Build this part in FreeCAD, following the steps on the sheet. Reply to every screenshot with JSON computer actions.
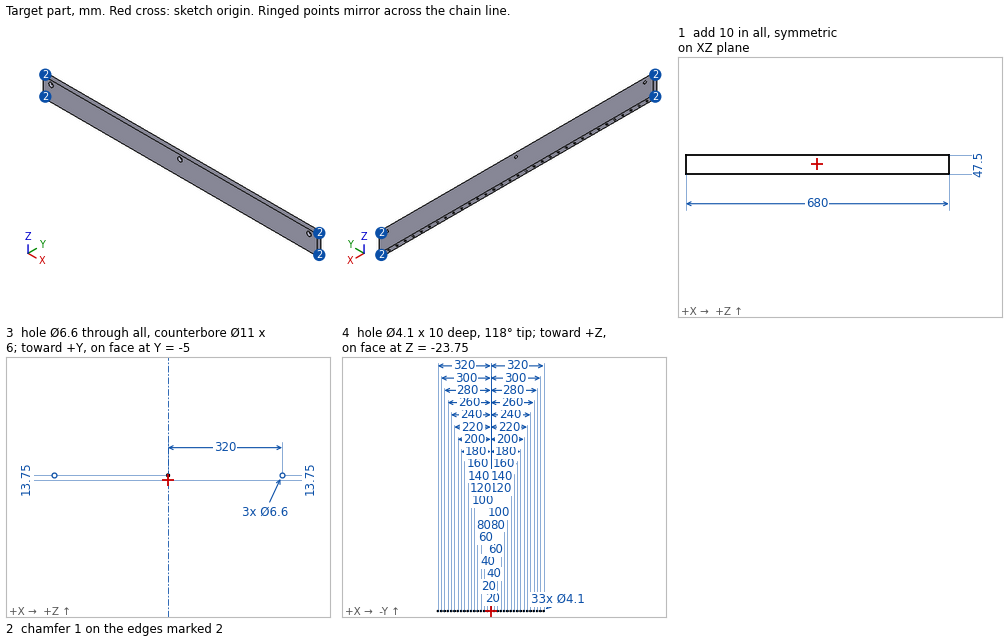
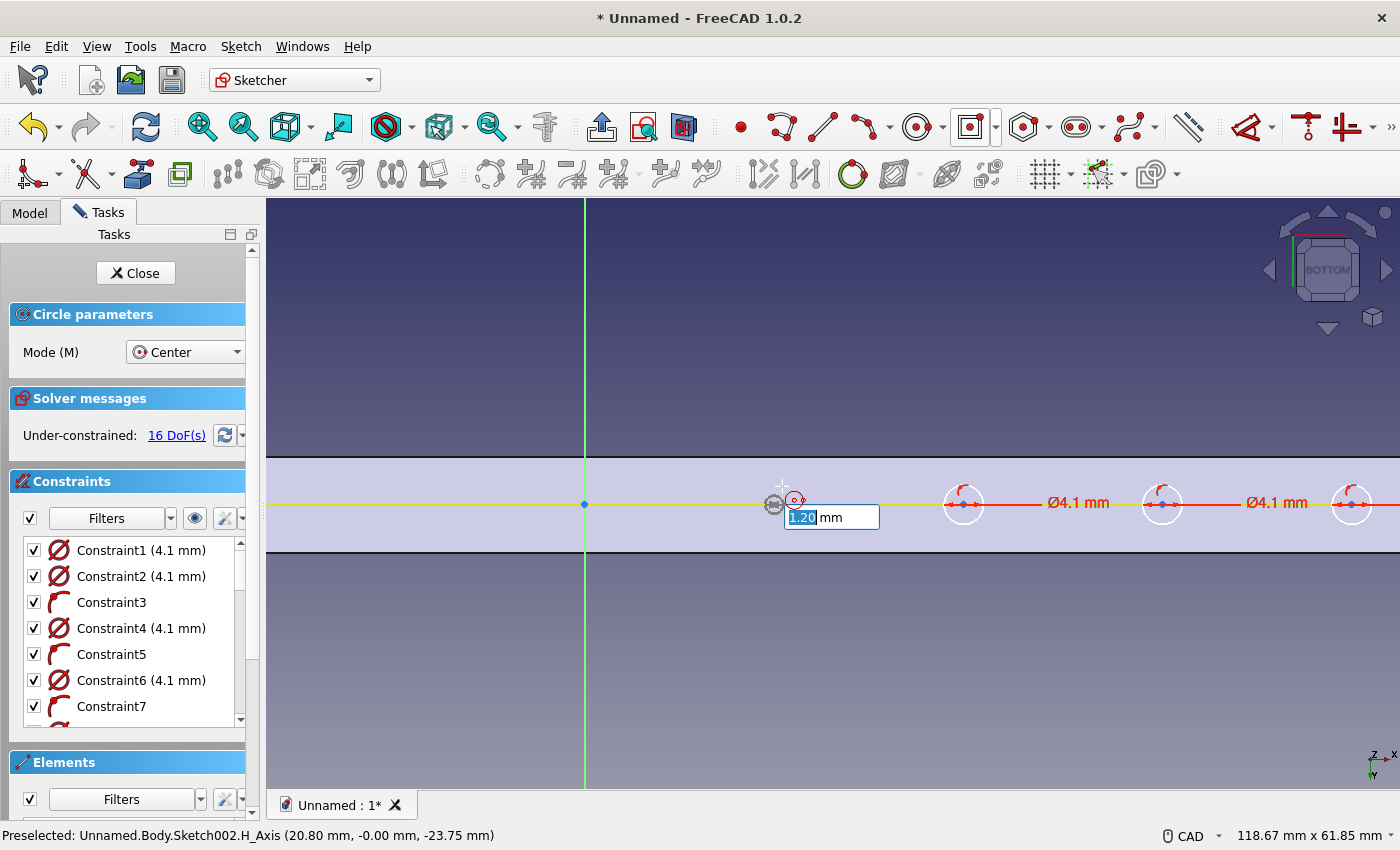
{"action": "type", "text": "4.1"}
{"action": "key", "text": "Return"}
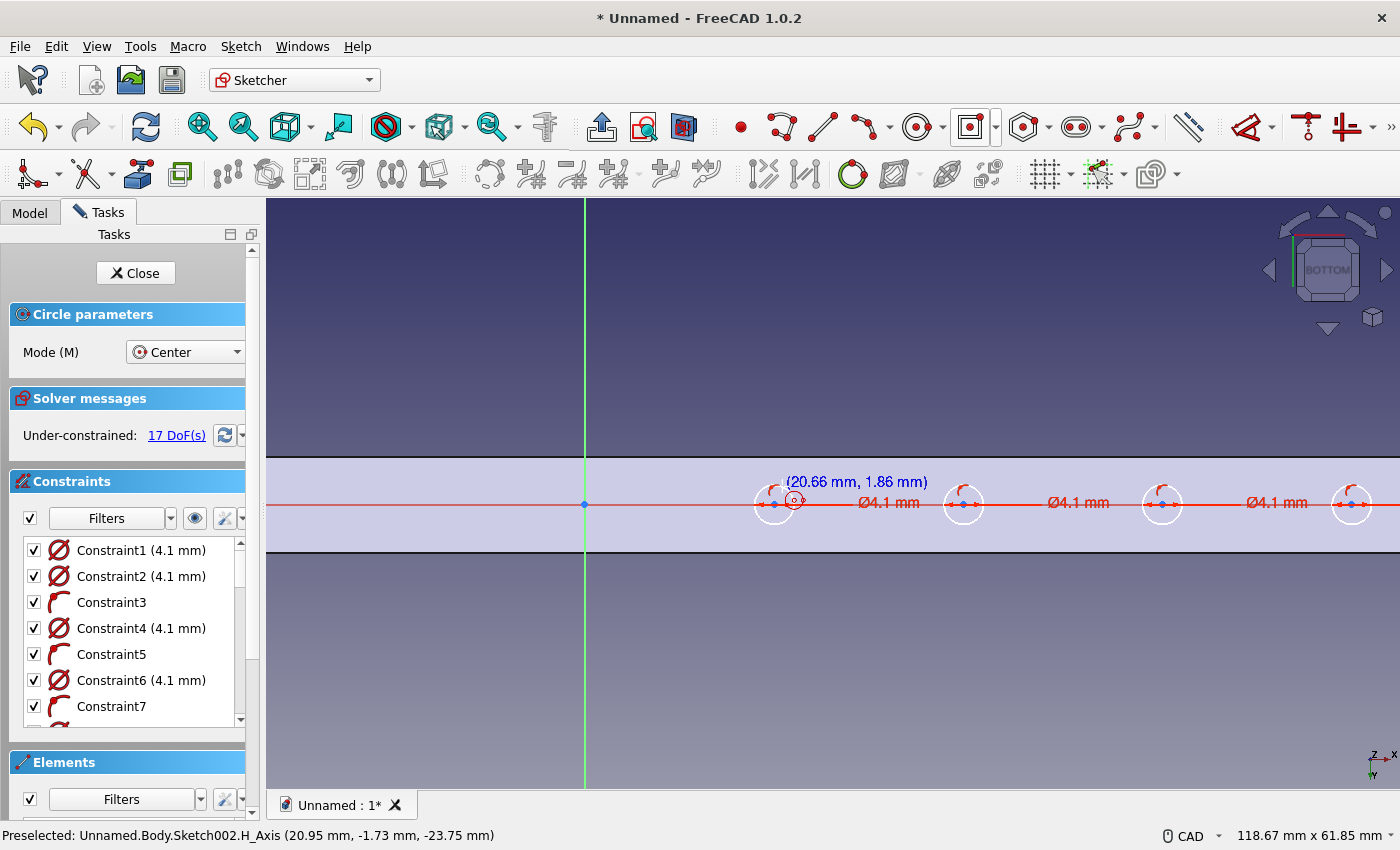
{"action": "scroll", "coordinate": [787, 492], "scroll_direction": "down", "scroll_amount": 11}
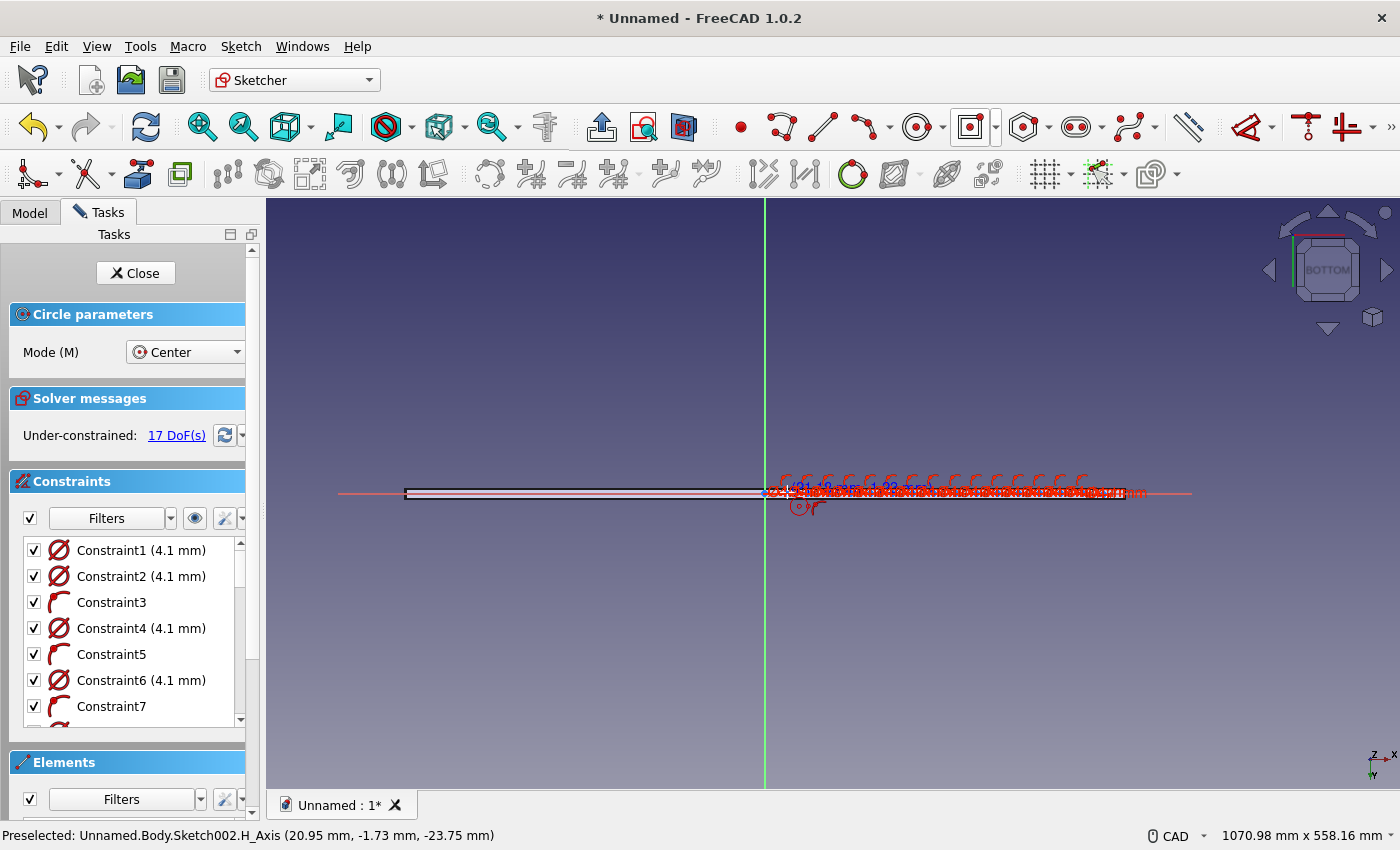
{"action": "left_click", "coordinate": [765, 494]}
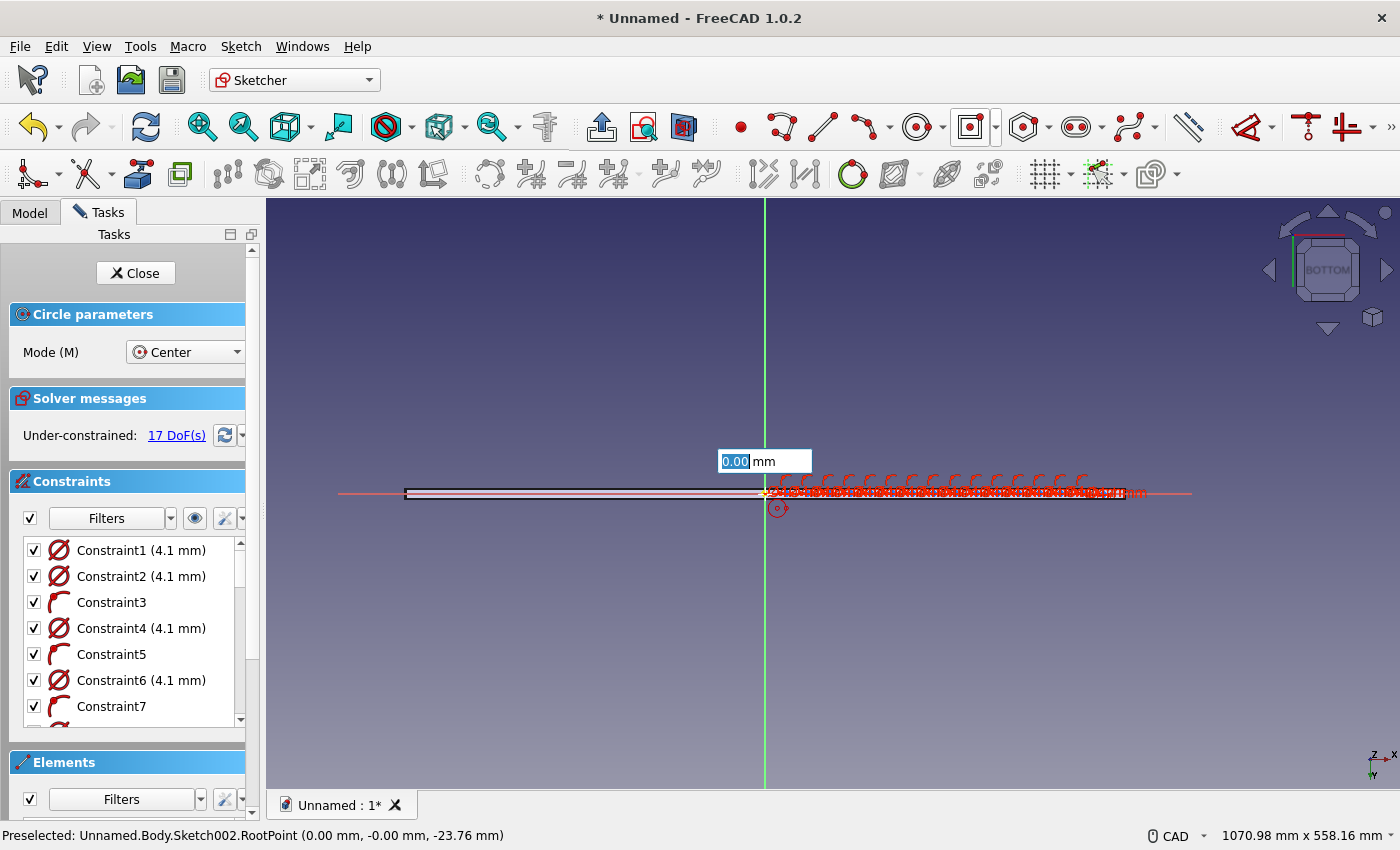
{"action": "scroll", "coordinate": [767, 492], "scroll_direction": "up", "scroll_amount": 12}
{"action": "mouse_move", "coordinate": [757, 491]}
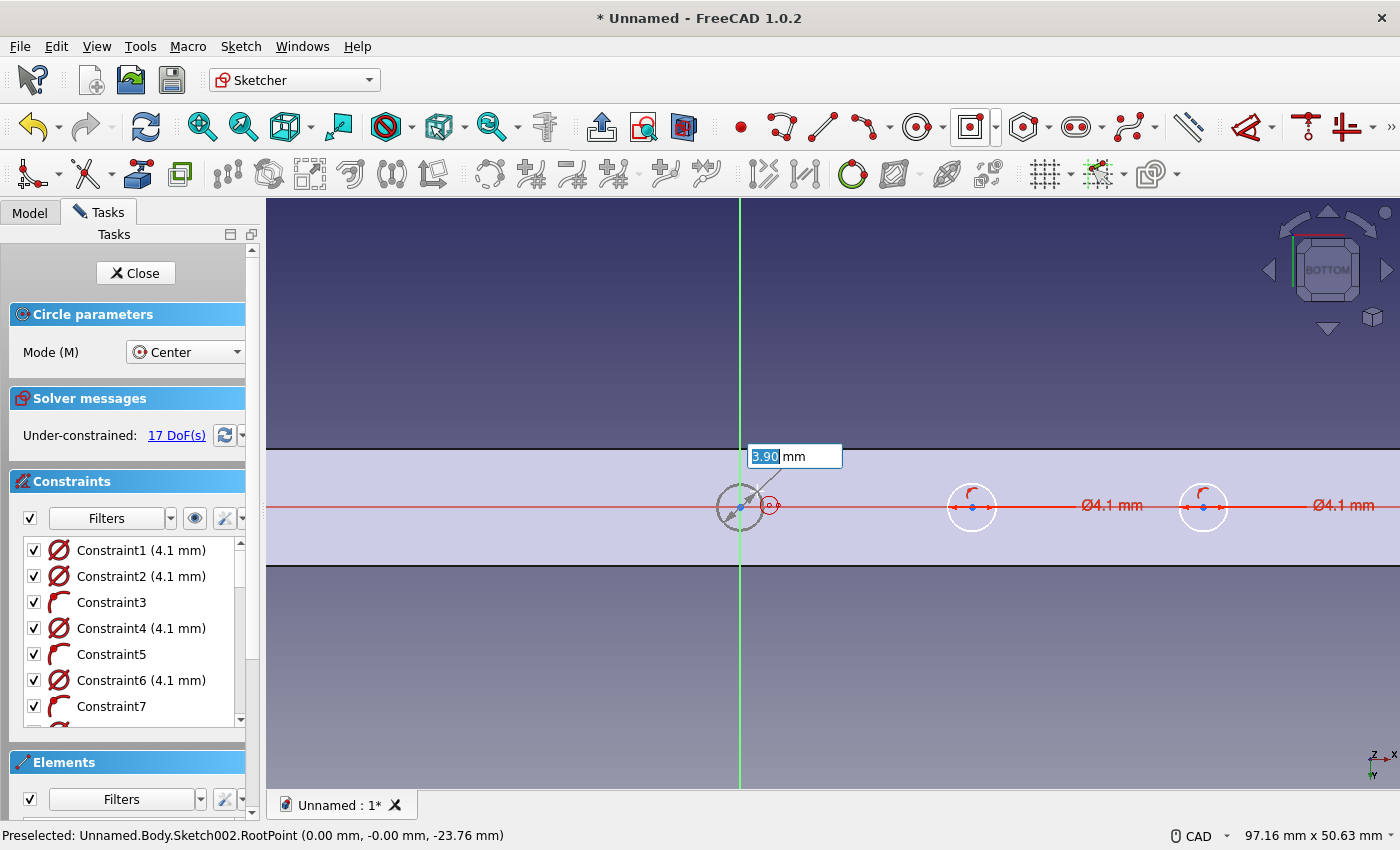
{"action": "type", "text": "4.1"}
{"action": "key", "text": "Return"}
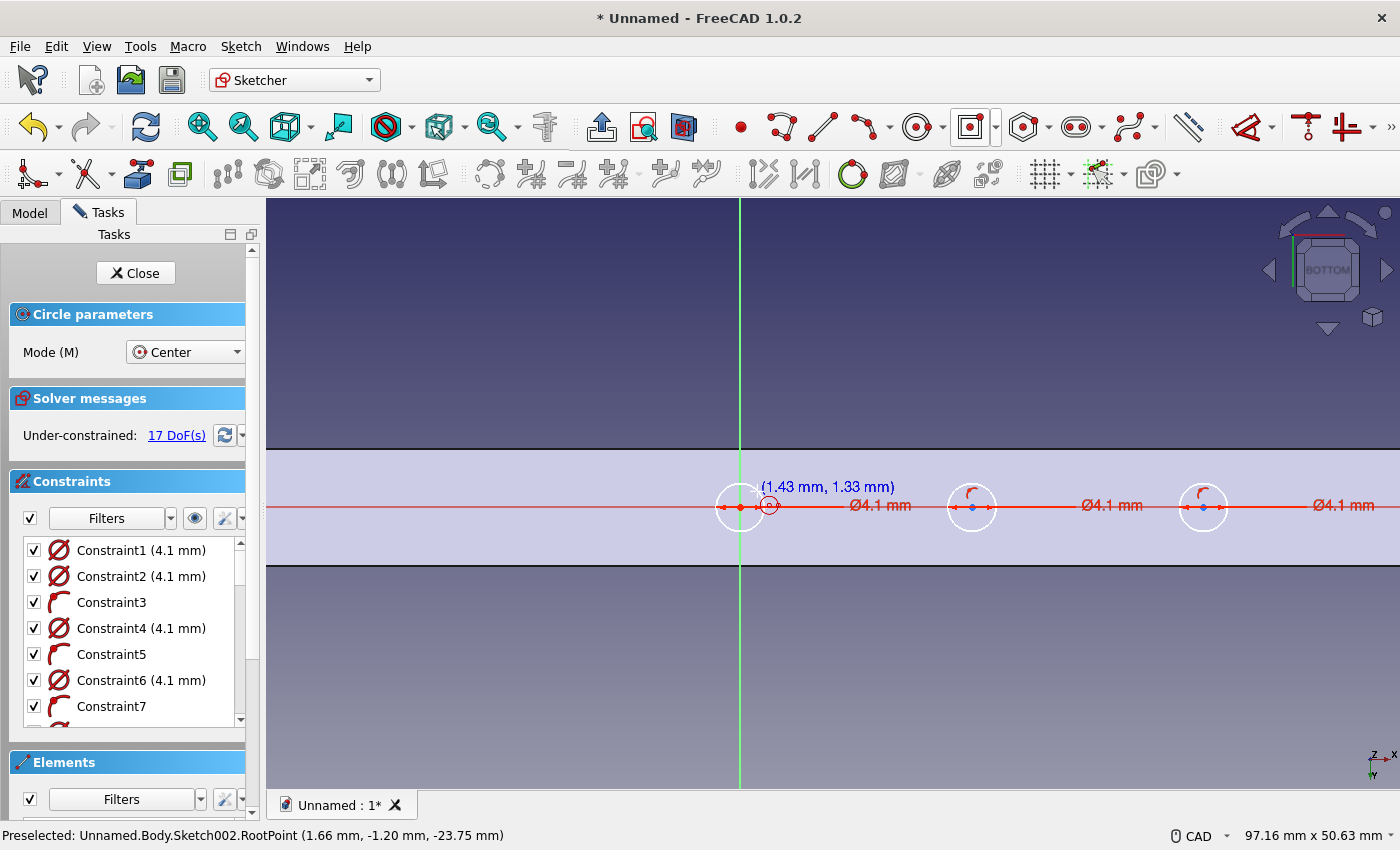
{"action": "scroll", "coordinate": [767, 492], "scroll_direction": "down", "scroll_amount": 12}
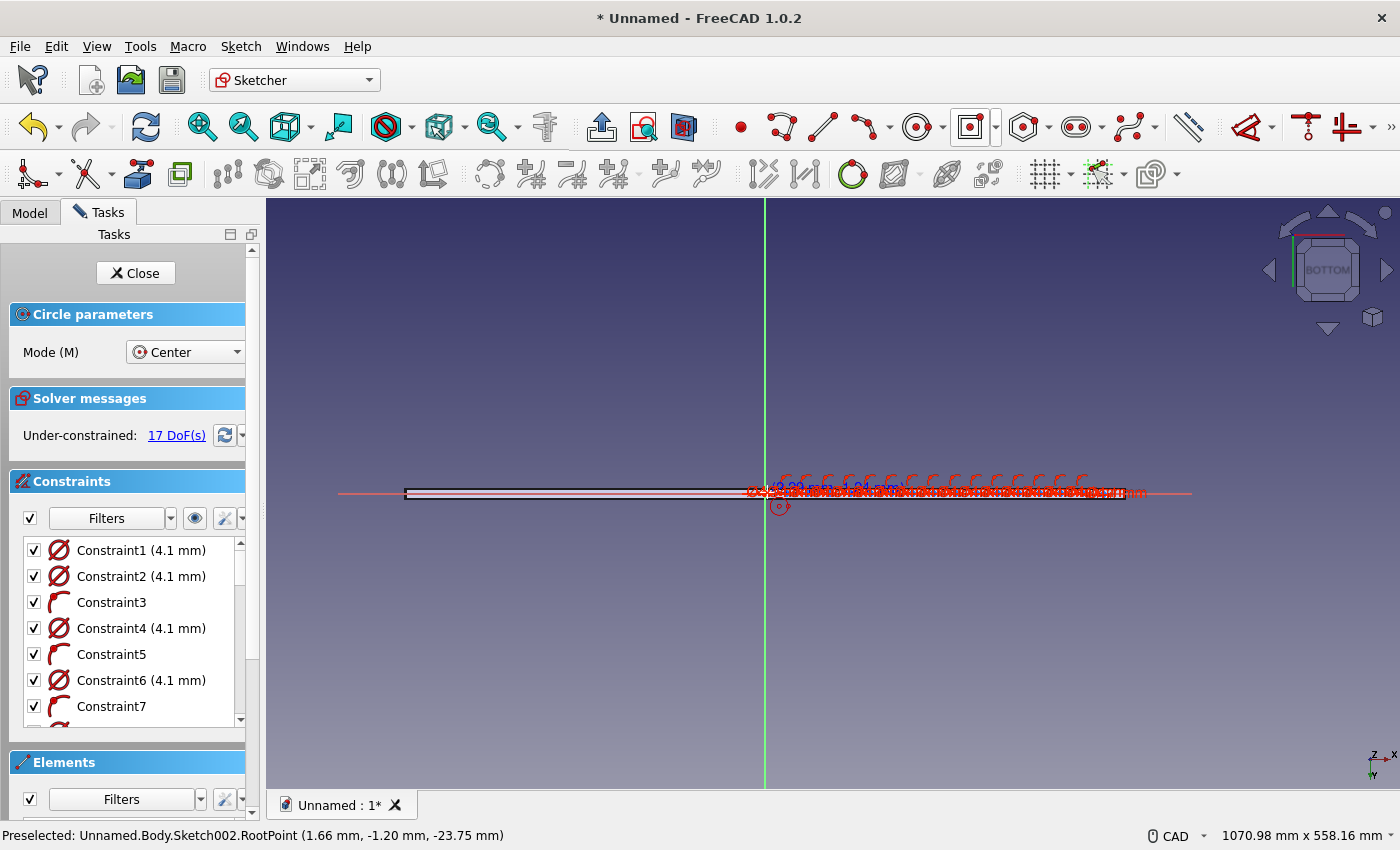
{"action": "left_click", "coordinate": [744, 494]}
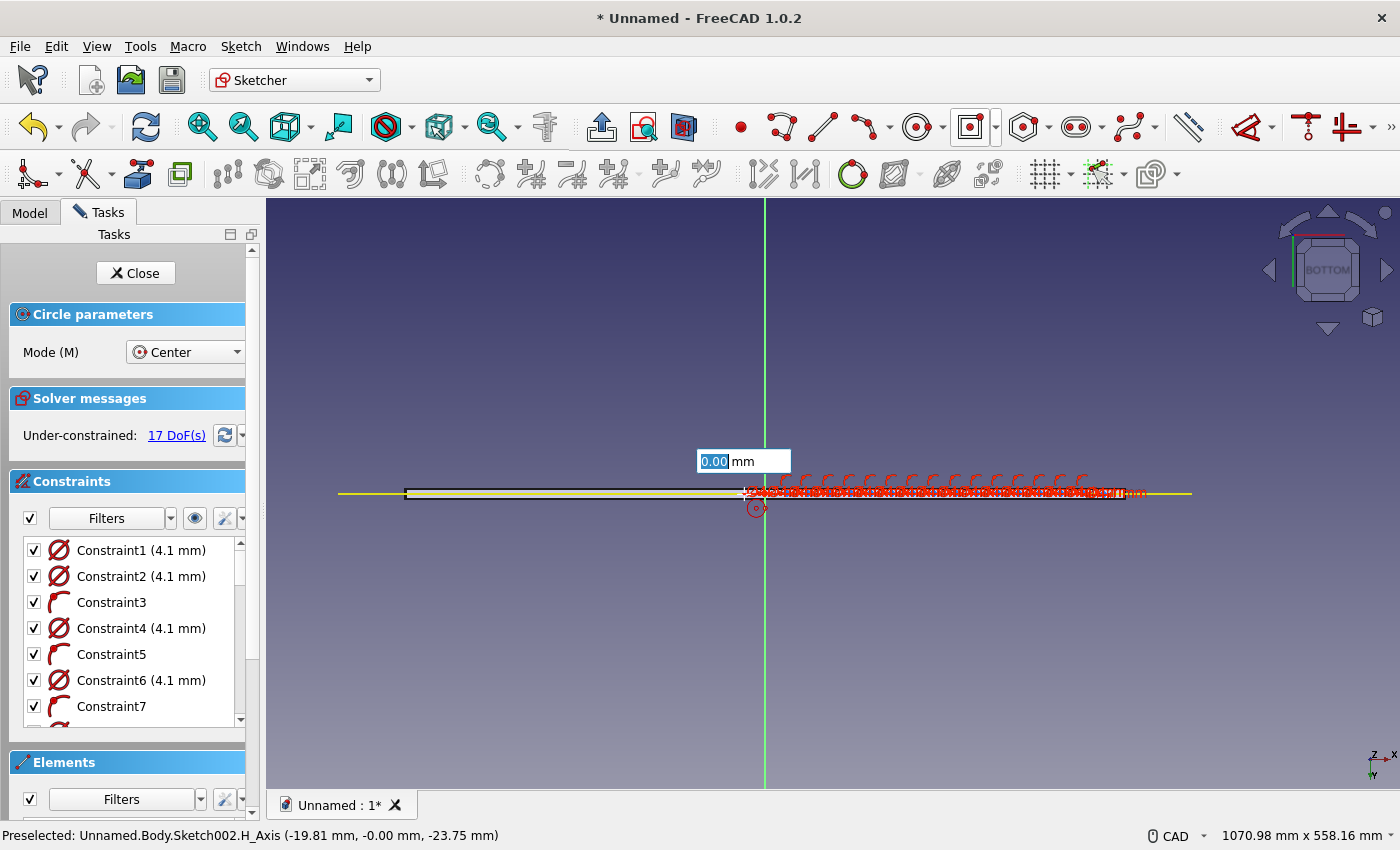
{"action": "scroll", "coordinate": [743, 496], "scroll_direction": "up", "scroll_amount": 11}
{"action": "mouse_move", "coordinate": [740, 491]}